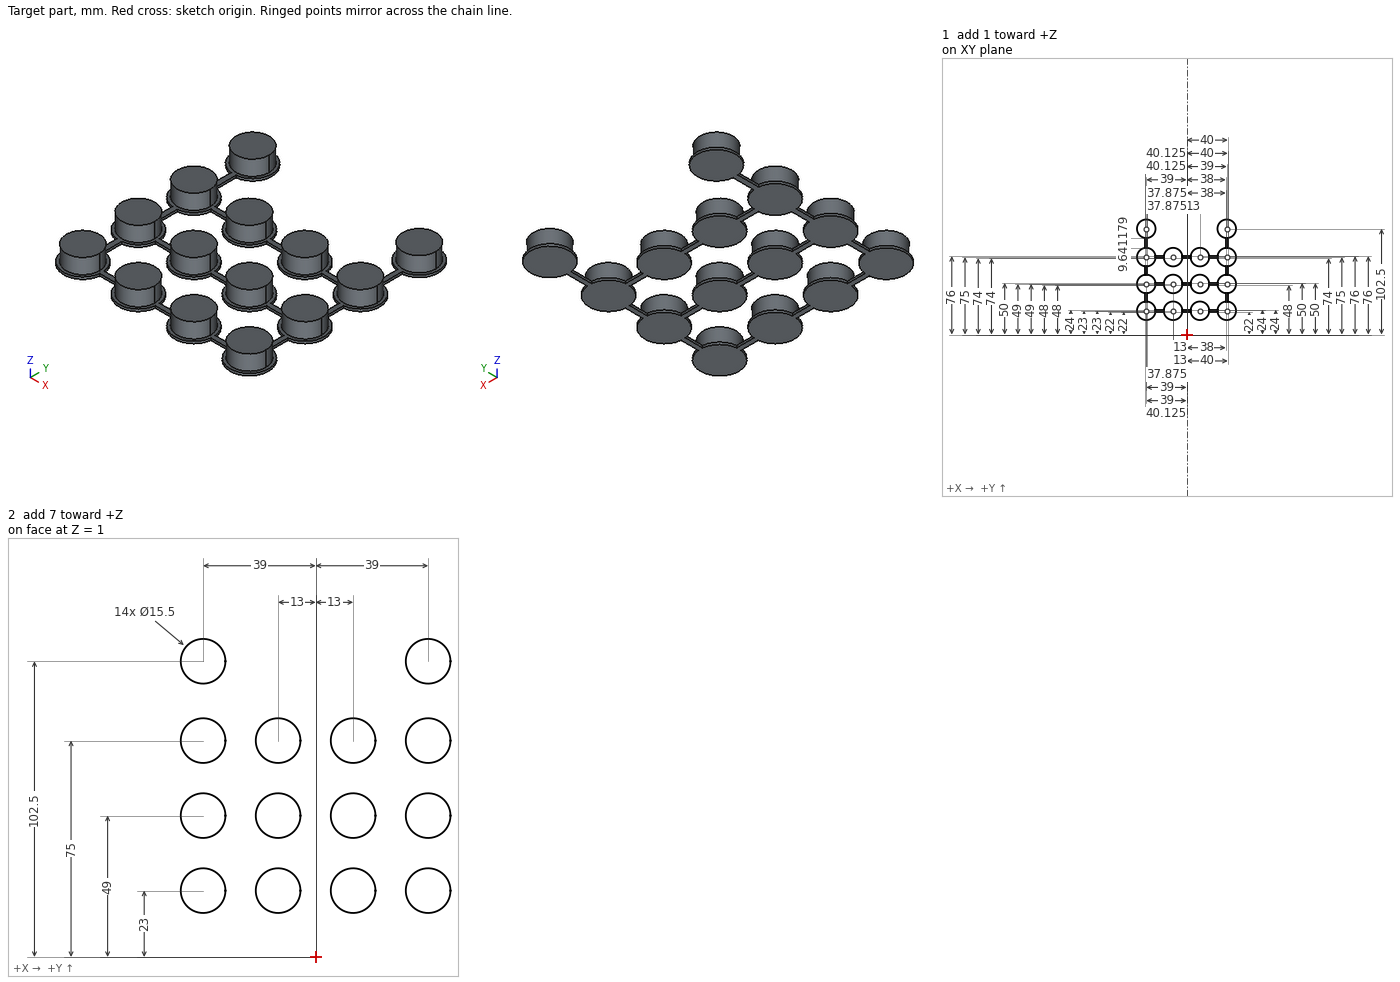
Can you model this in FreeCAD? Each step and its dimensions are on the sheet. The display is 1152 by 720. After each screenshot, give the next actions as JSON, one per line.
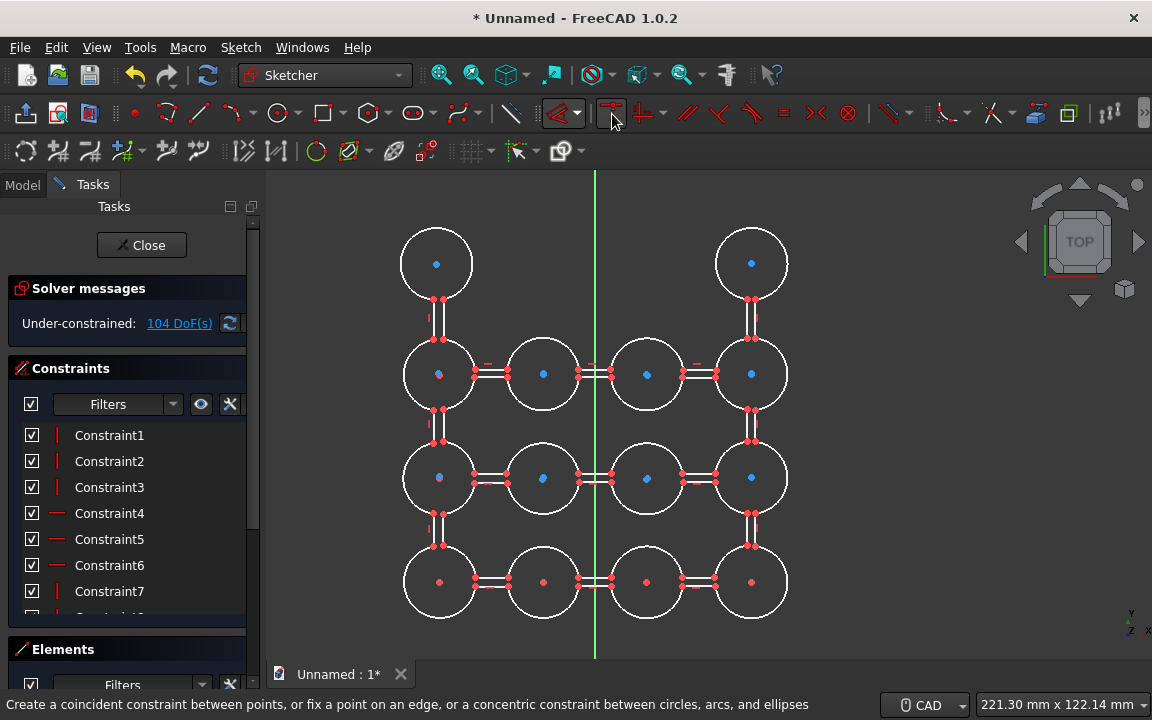
{"action": "left_click", "coordinate": [563, 344]}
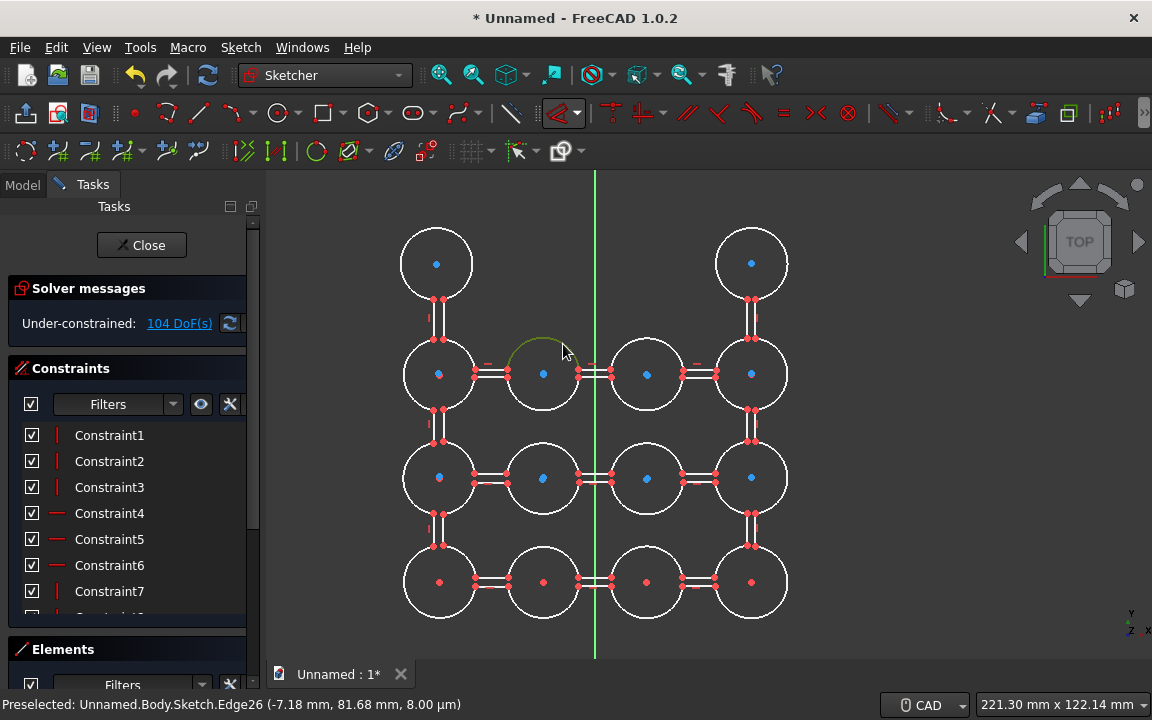
{"action": "left_click", "coordinate": [523, 404]}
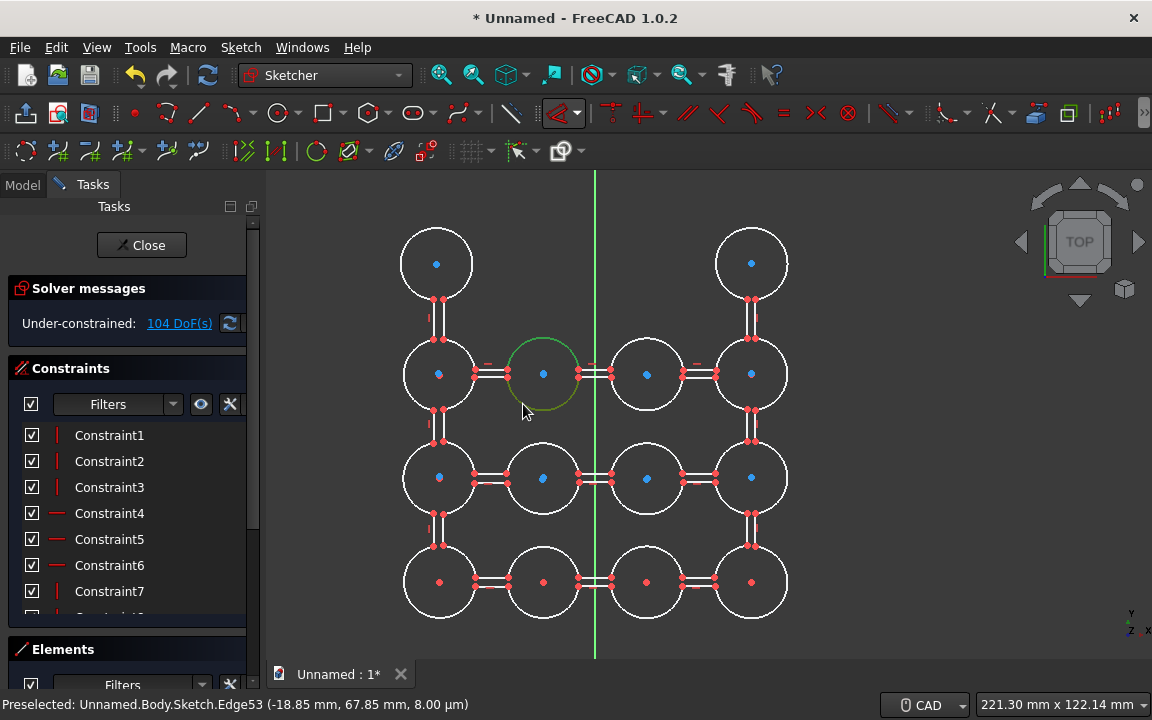
{"action": "left_click", "coordinate": [612, 114]}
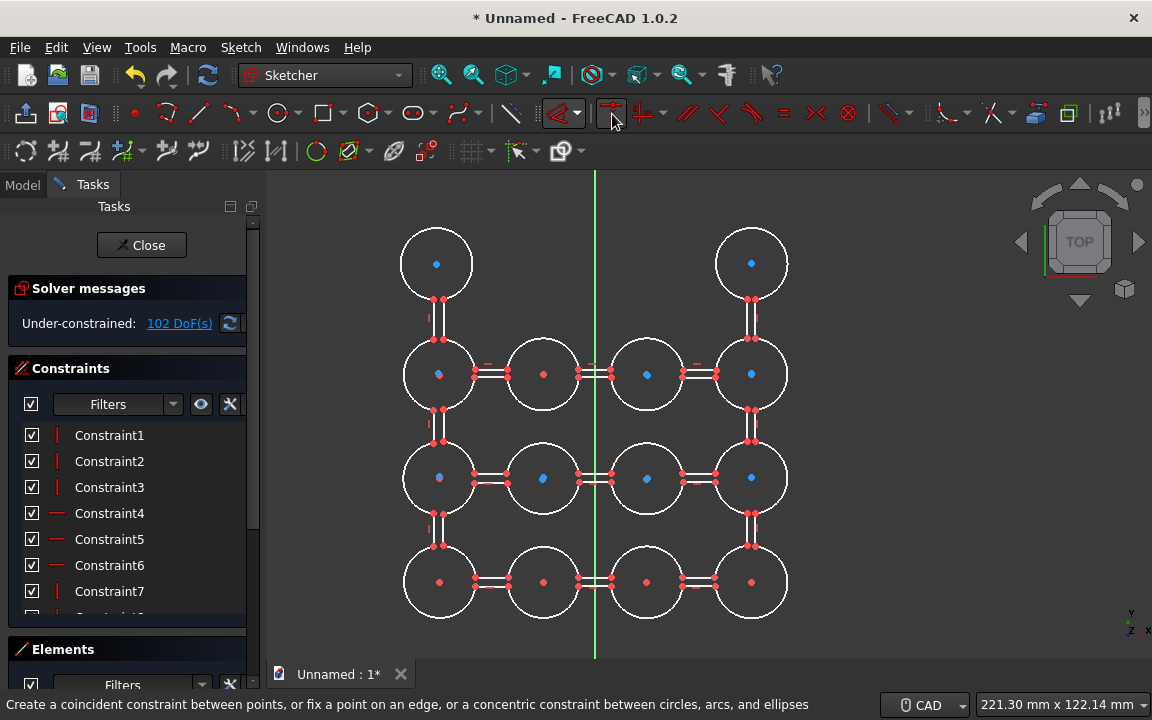
{"action": "left_click", "coordinate": [667, 344]}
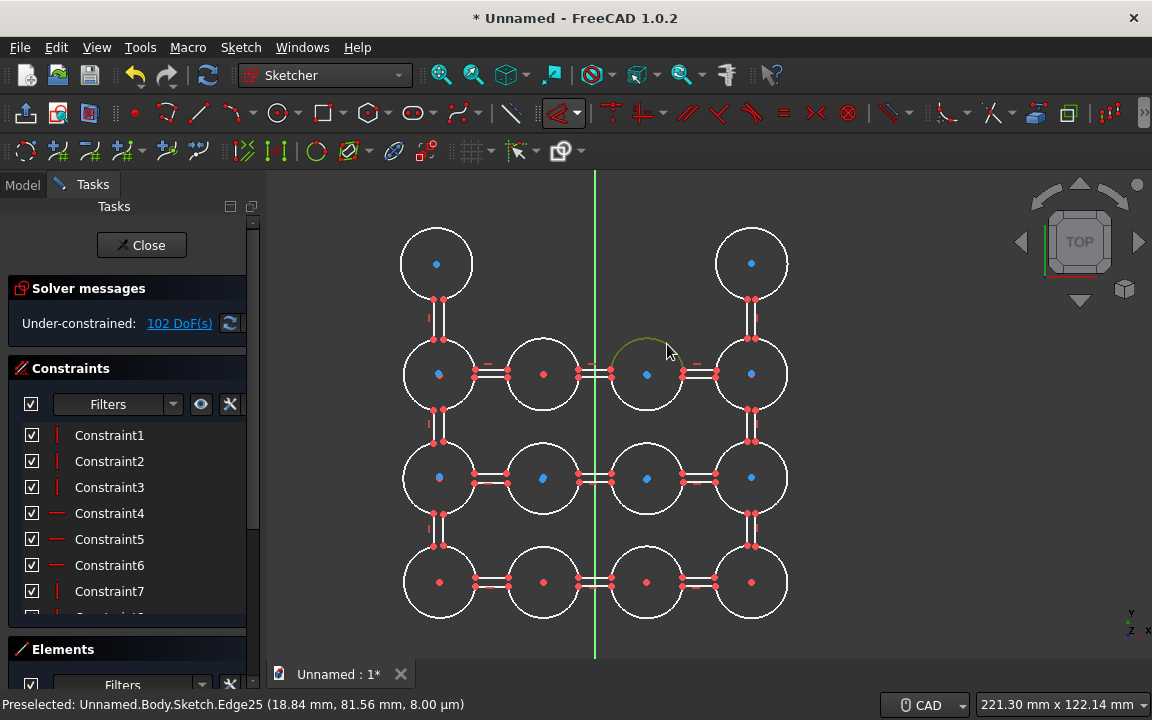
{"action": "left_click", "coordinate": [627, 404]}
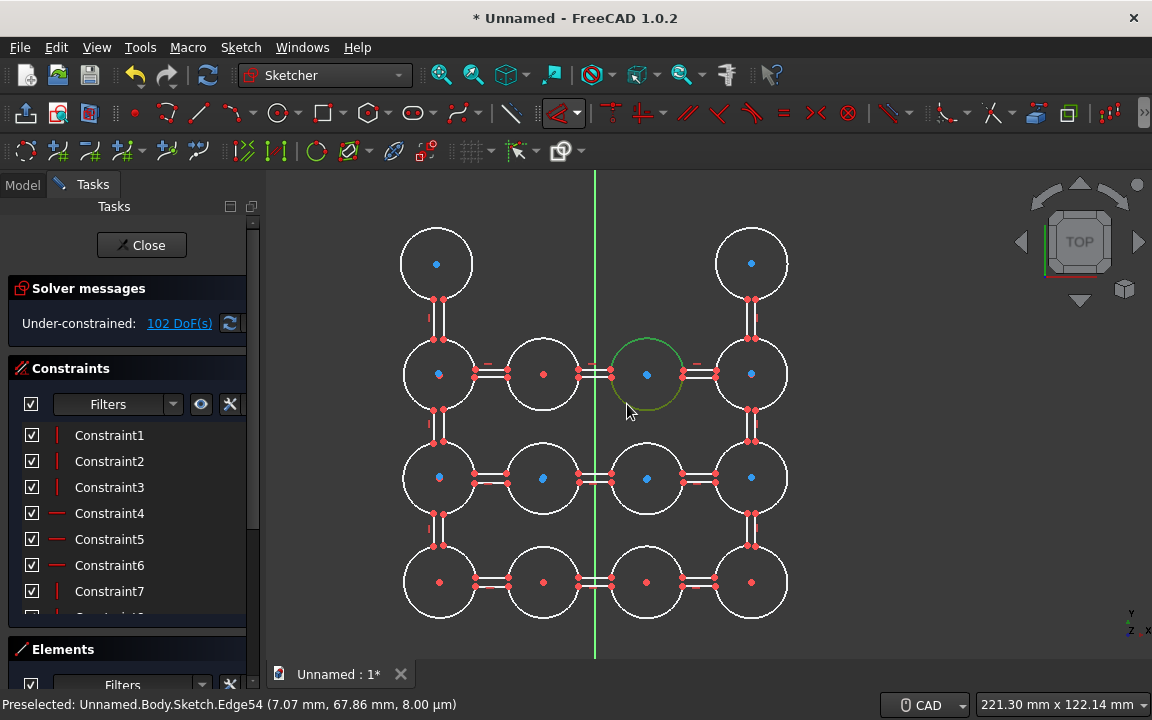
{"action": "left_click", "coordinate": [612, 114]}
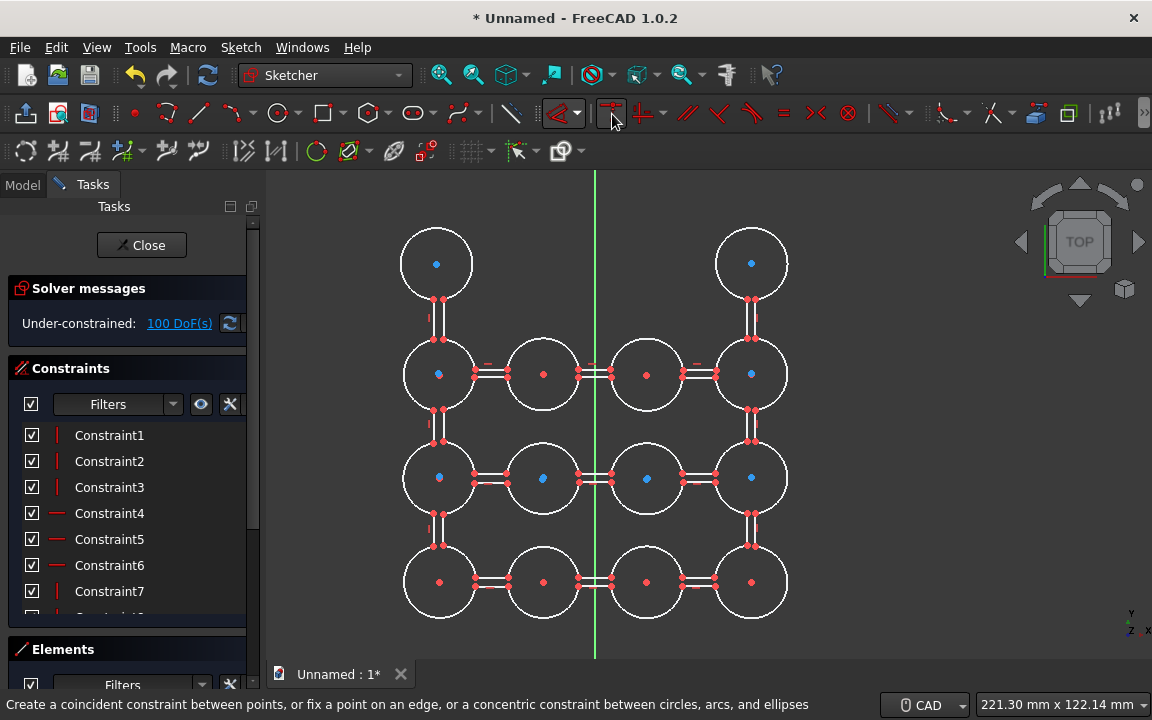
{"action": "left_click", "coordinate": [781, 394]}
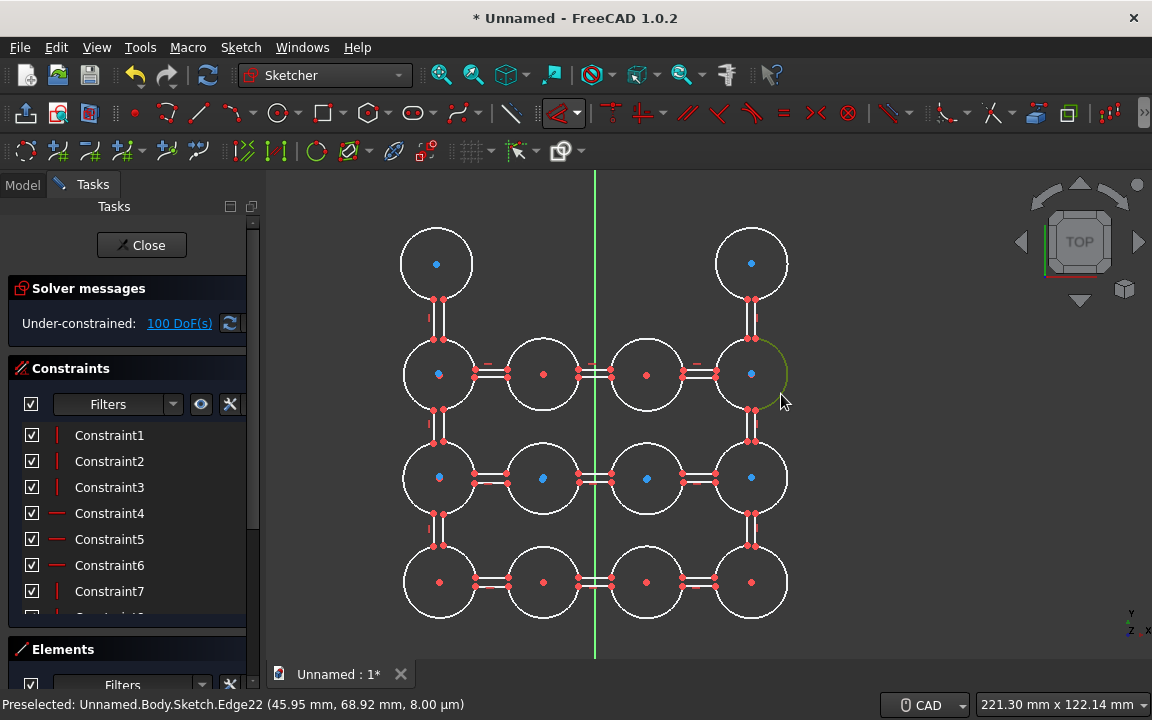
{"action": "left_click", "coordinate": [720, 391]}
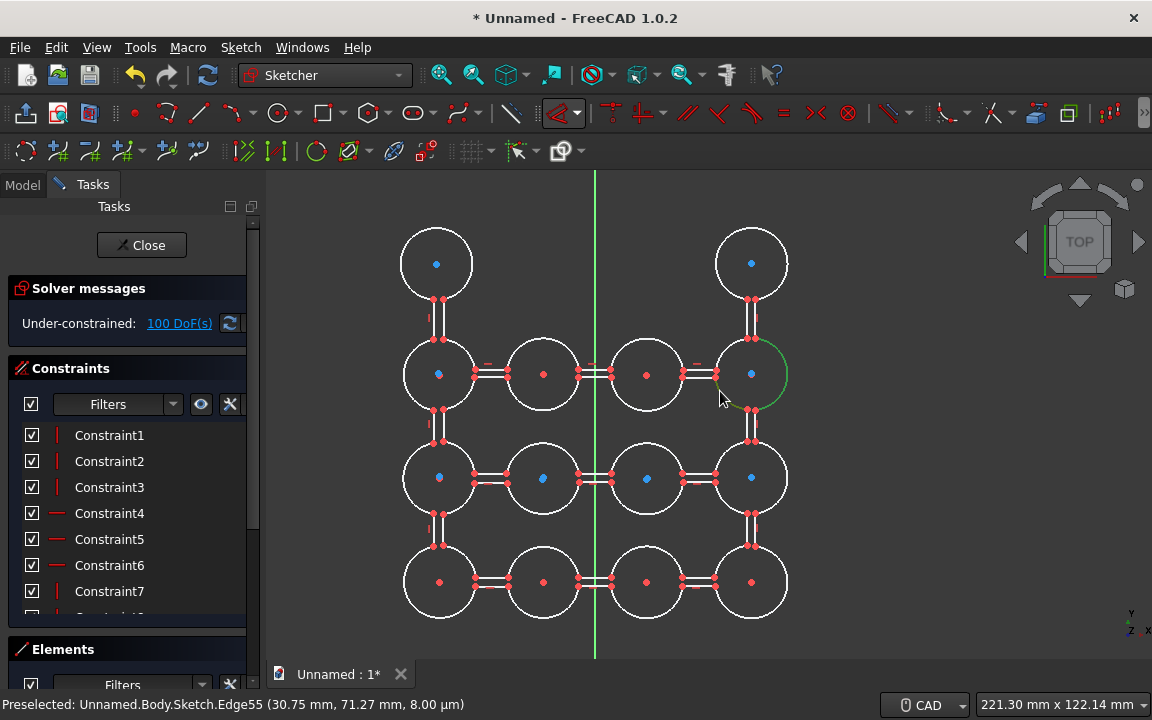
{"action": "left_click", "coordinate": [612, 114]}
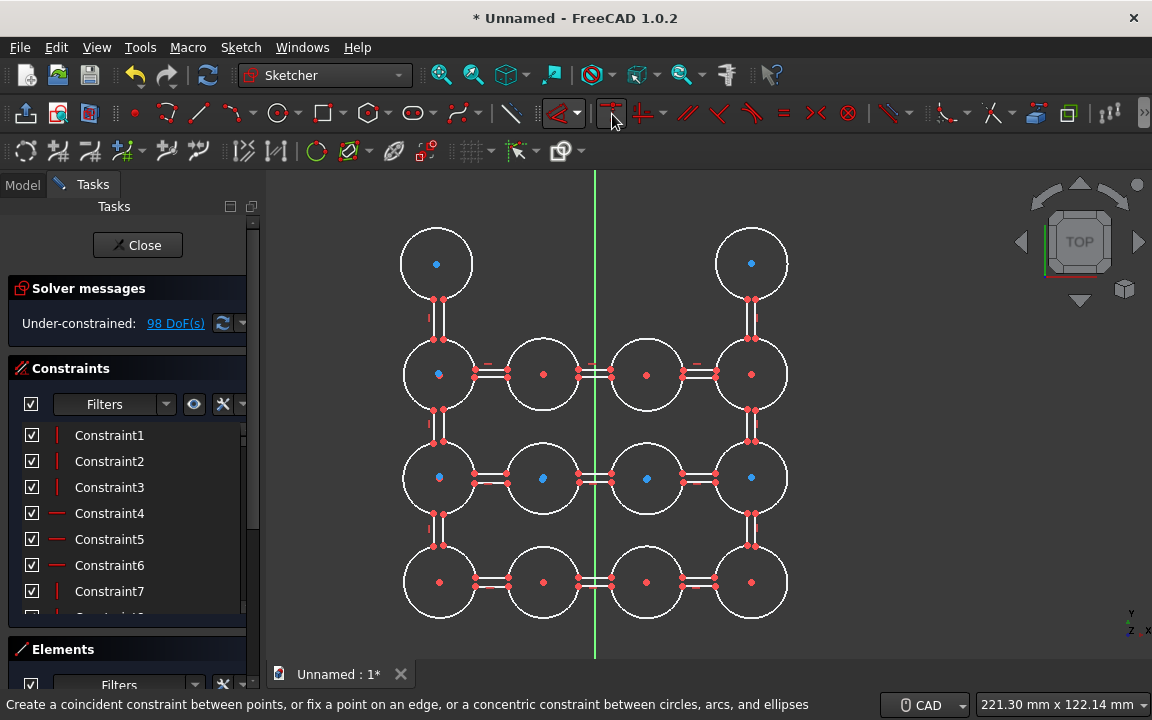
{"action": "left_click", "coordinate": [781, 498]}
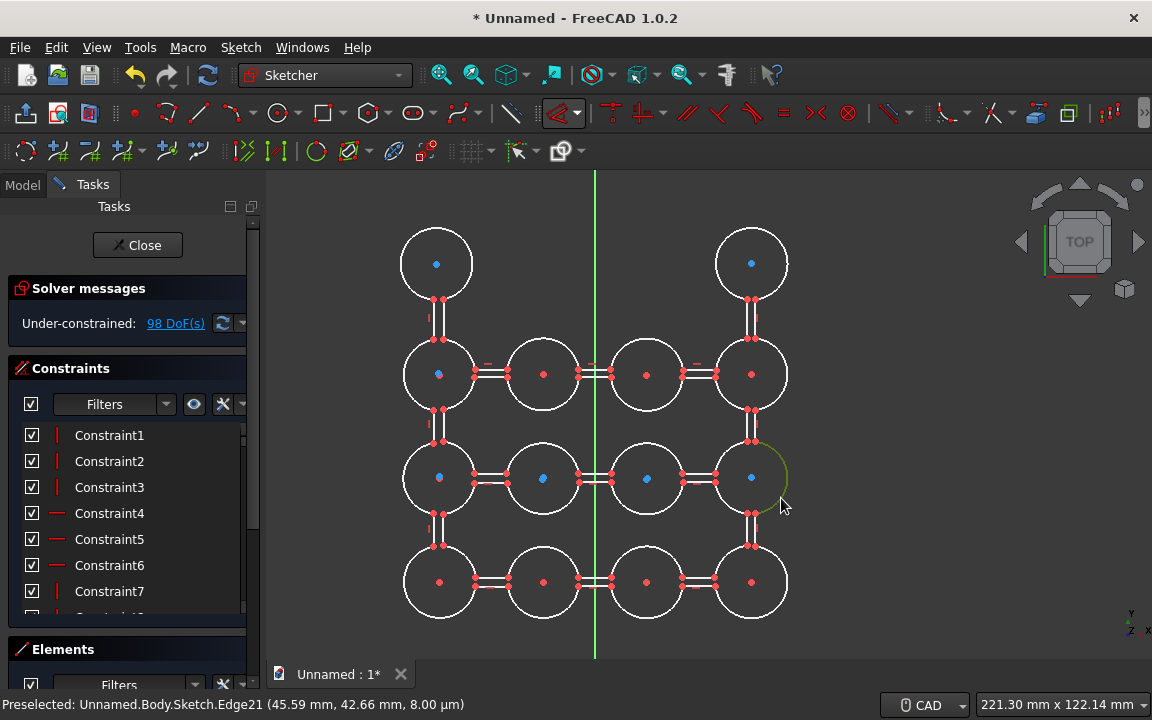
{"action": "left_click", "coordinate": [734, 446]}